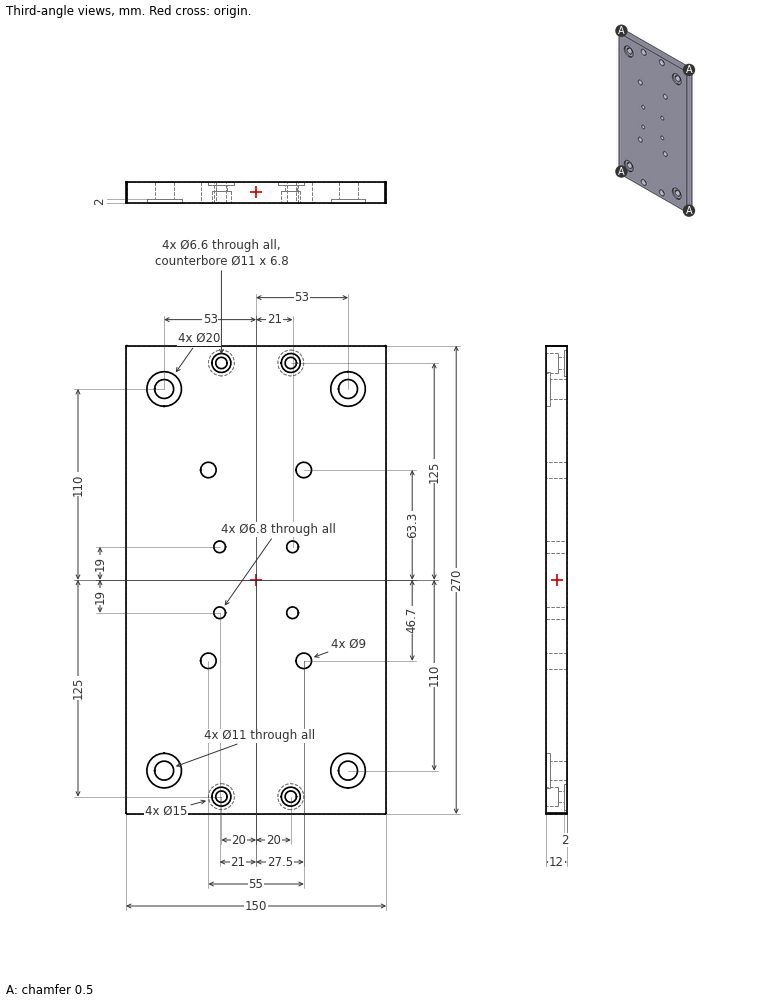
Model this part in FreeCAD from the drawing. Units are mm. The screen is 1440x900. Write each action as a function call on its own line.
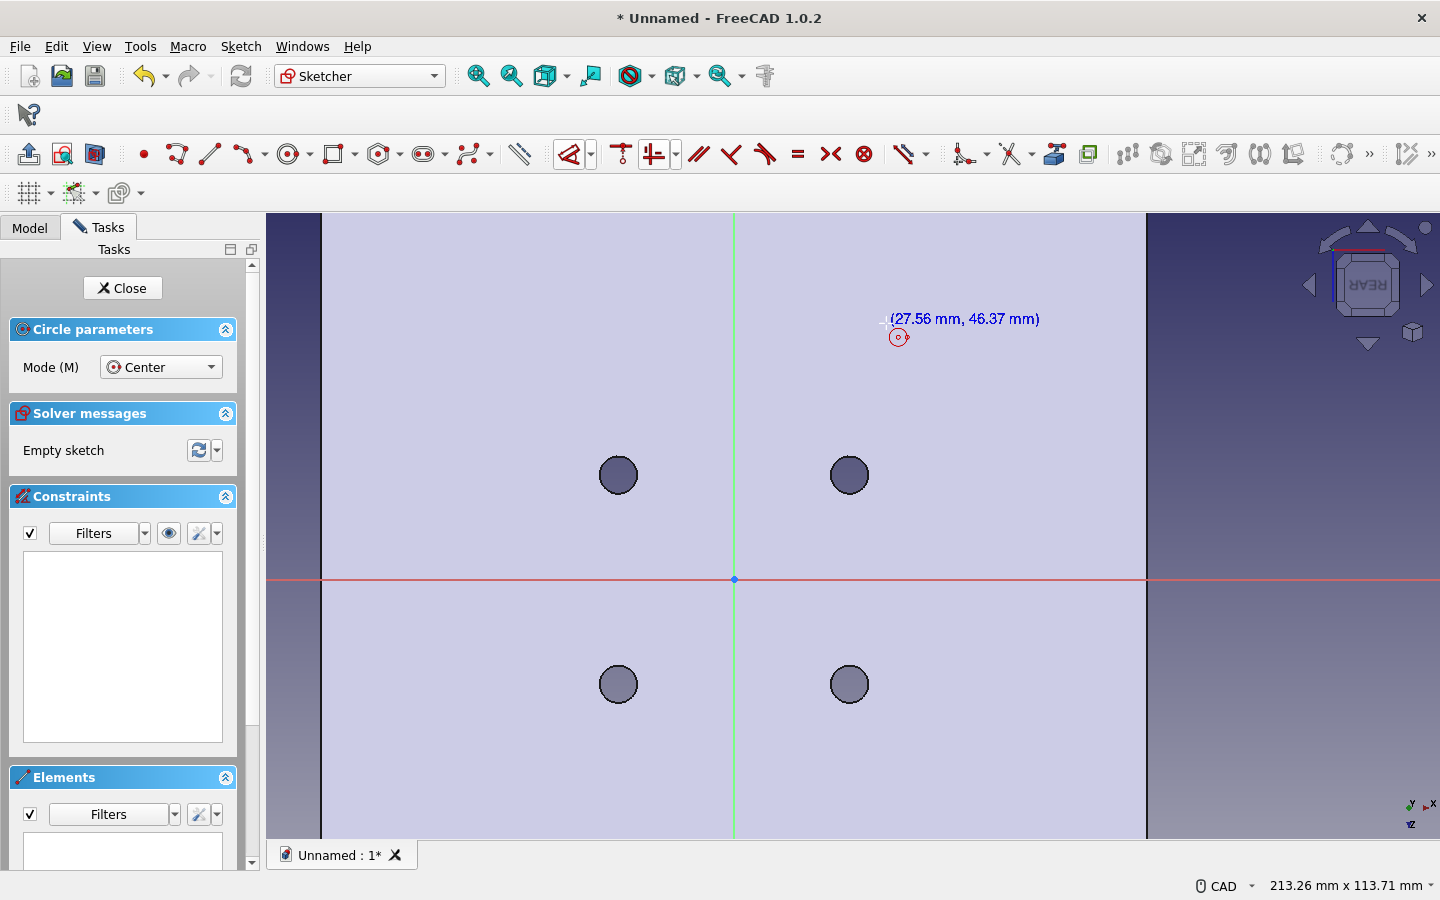
click(885, 323)
click(903, 305)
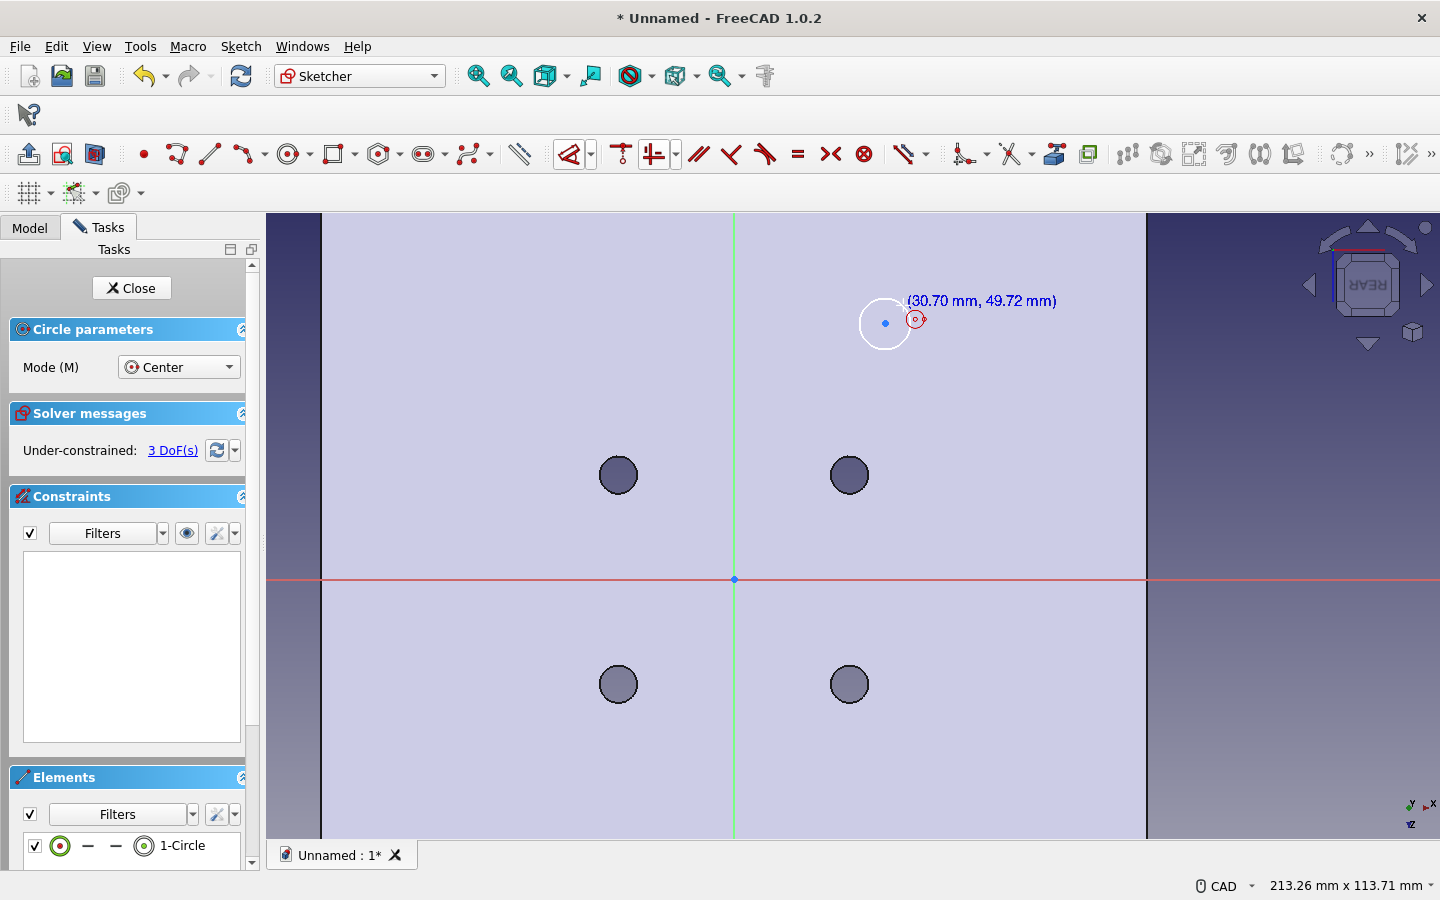
click(583, 323)
click(600, 305)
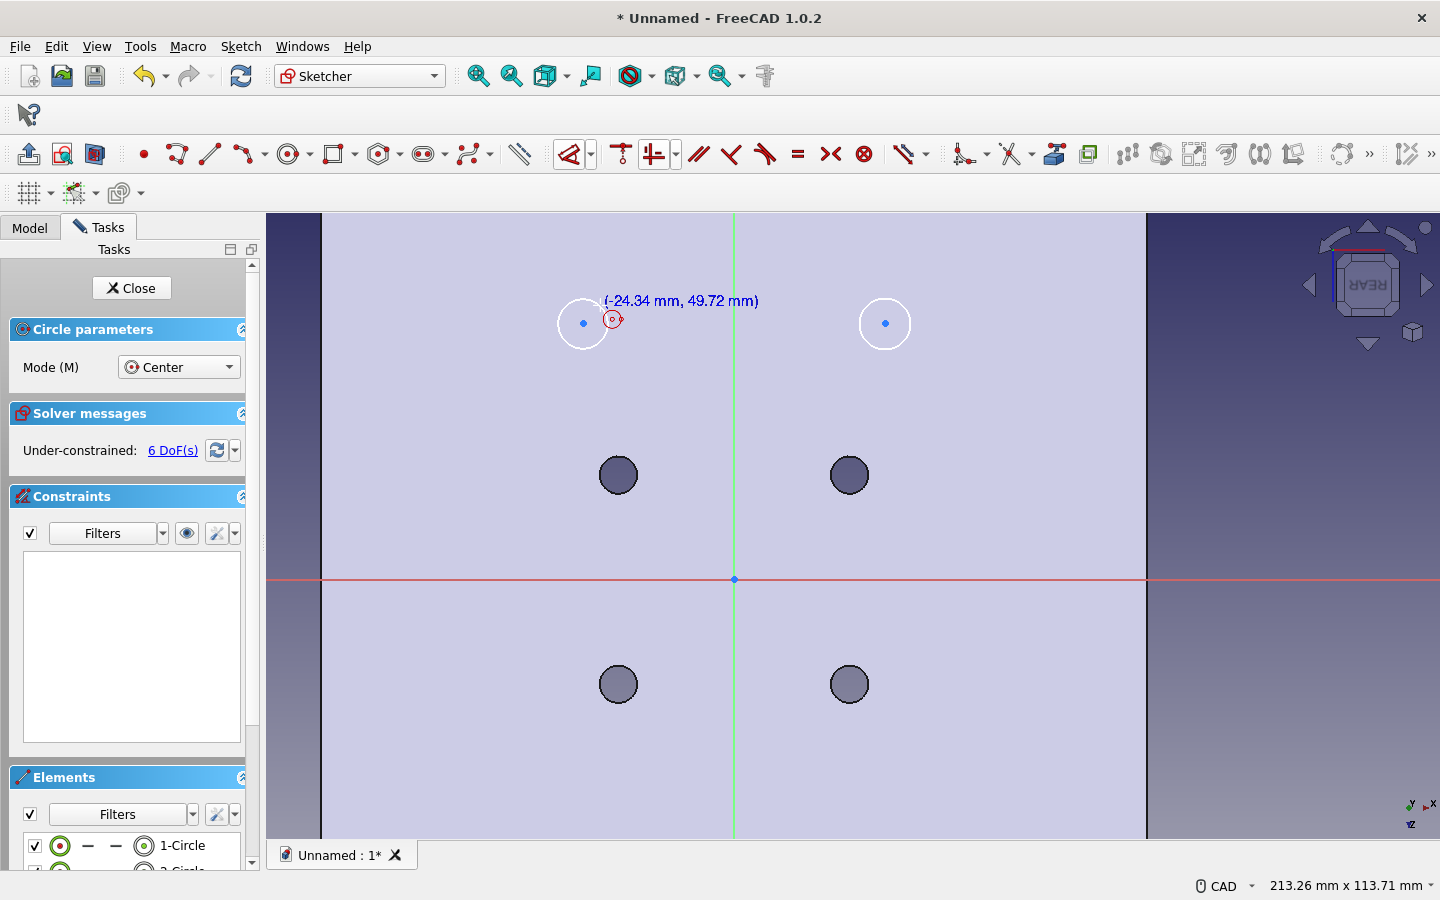
scroll(887, 324, down, 2)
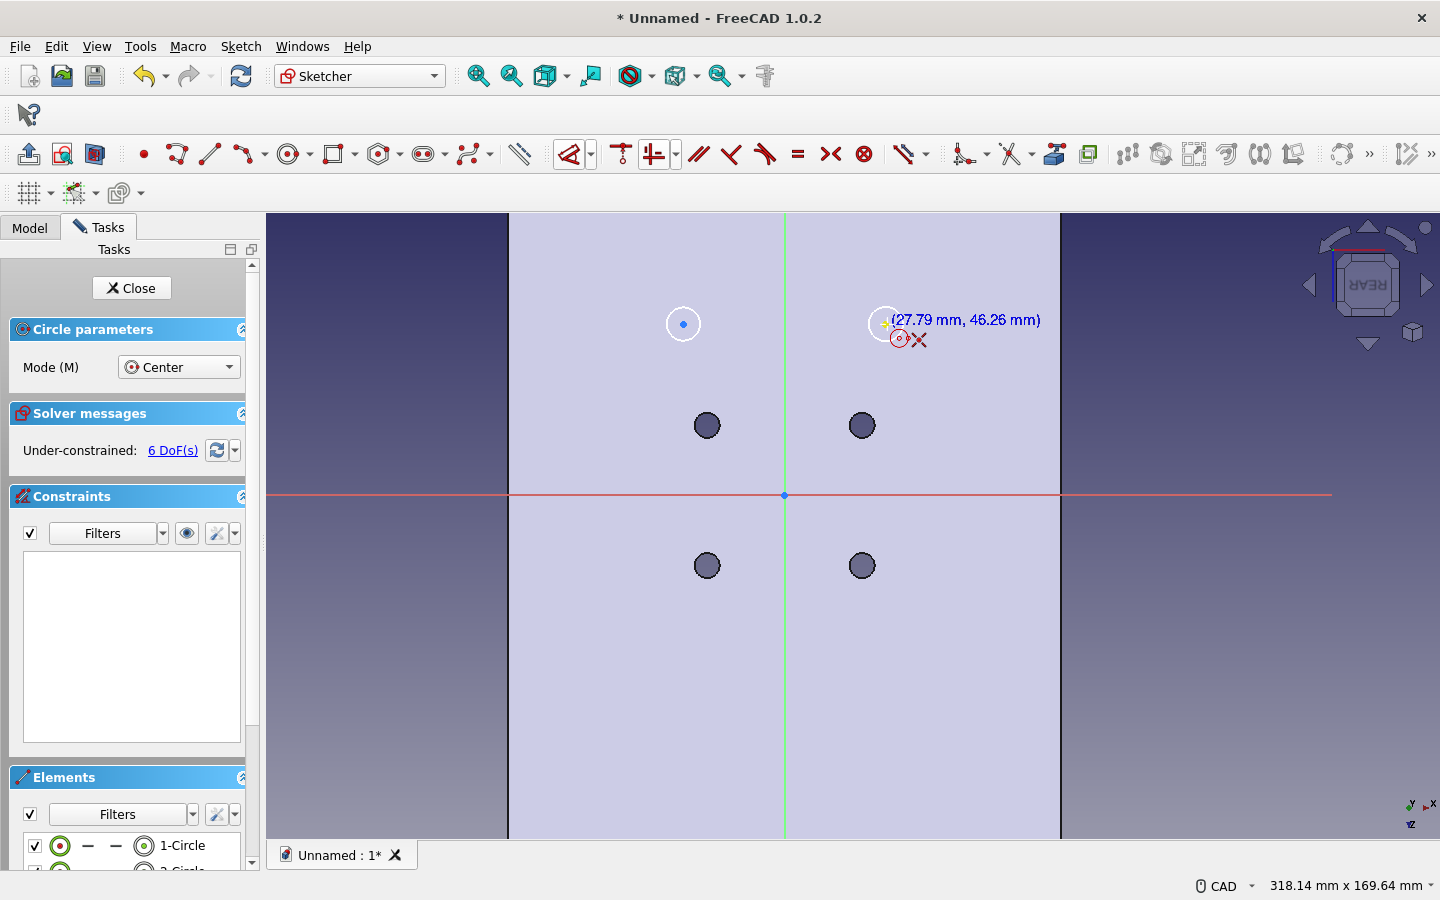
scroll(886, 729, up, 2)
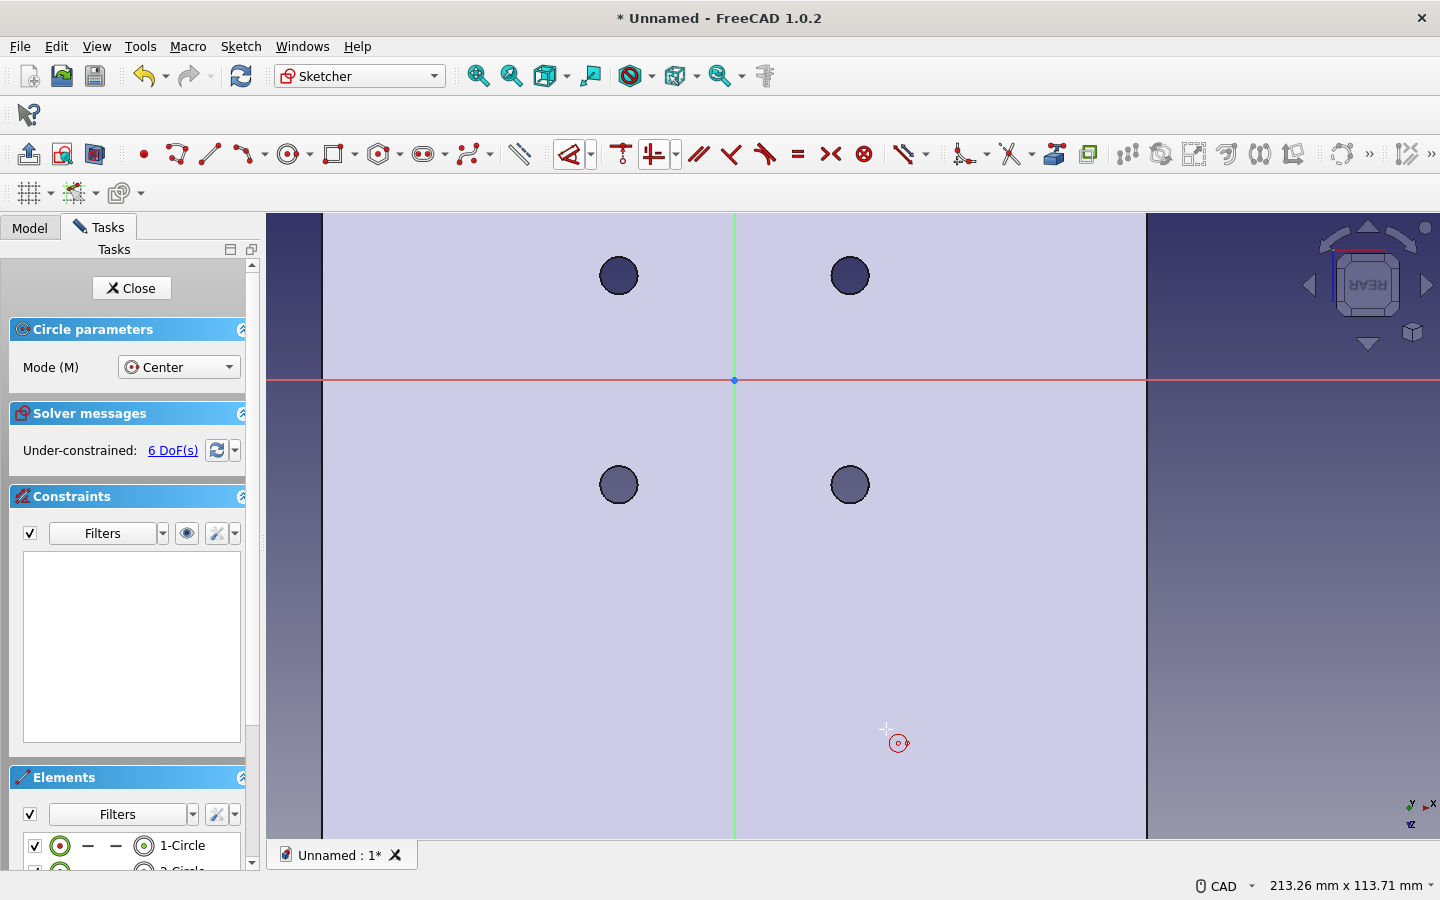
click(886, 729)
click(903, 711)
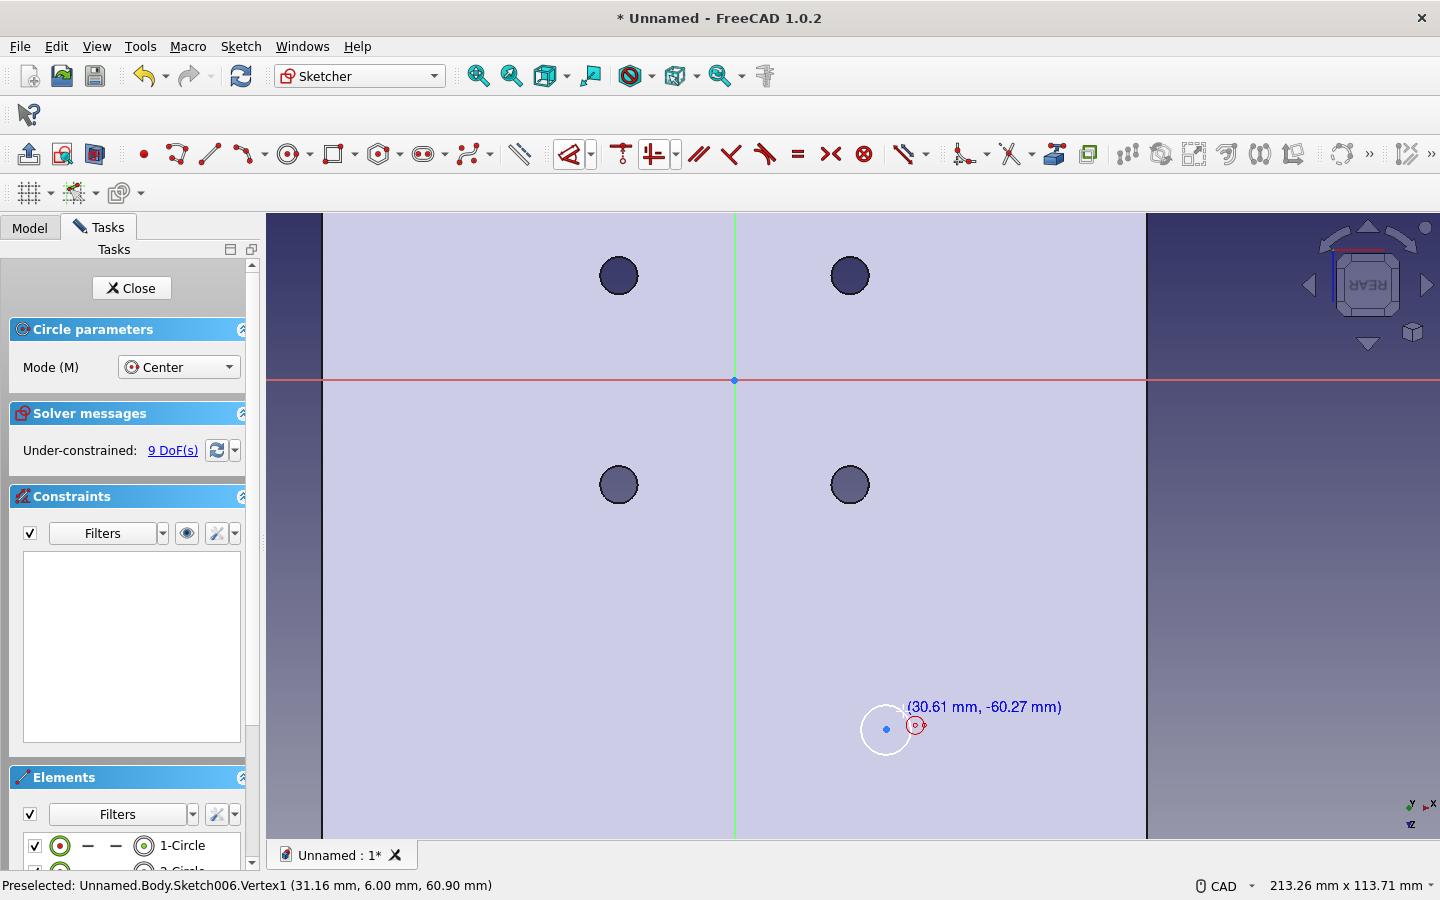
click(583, 729)
click(601, 711)
key(Escape)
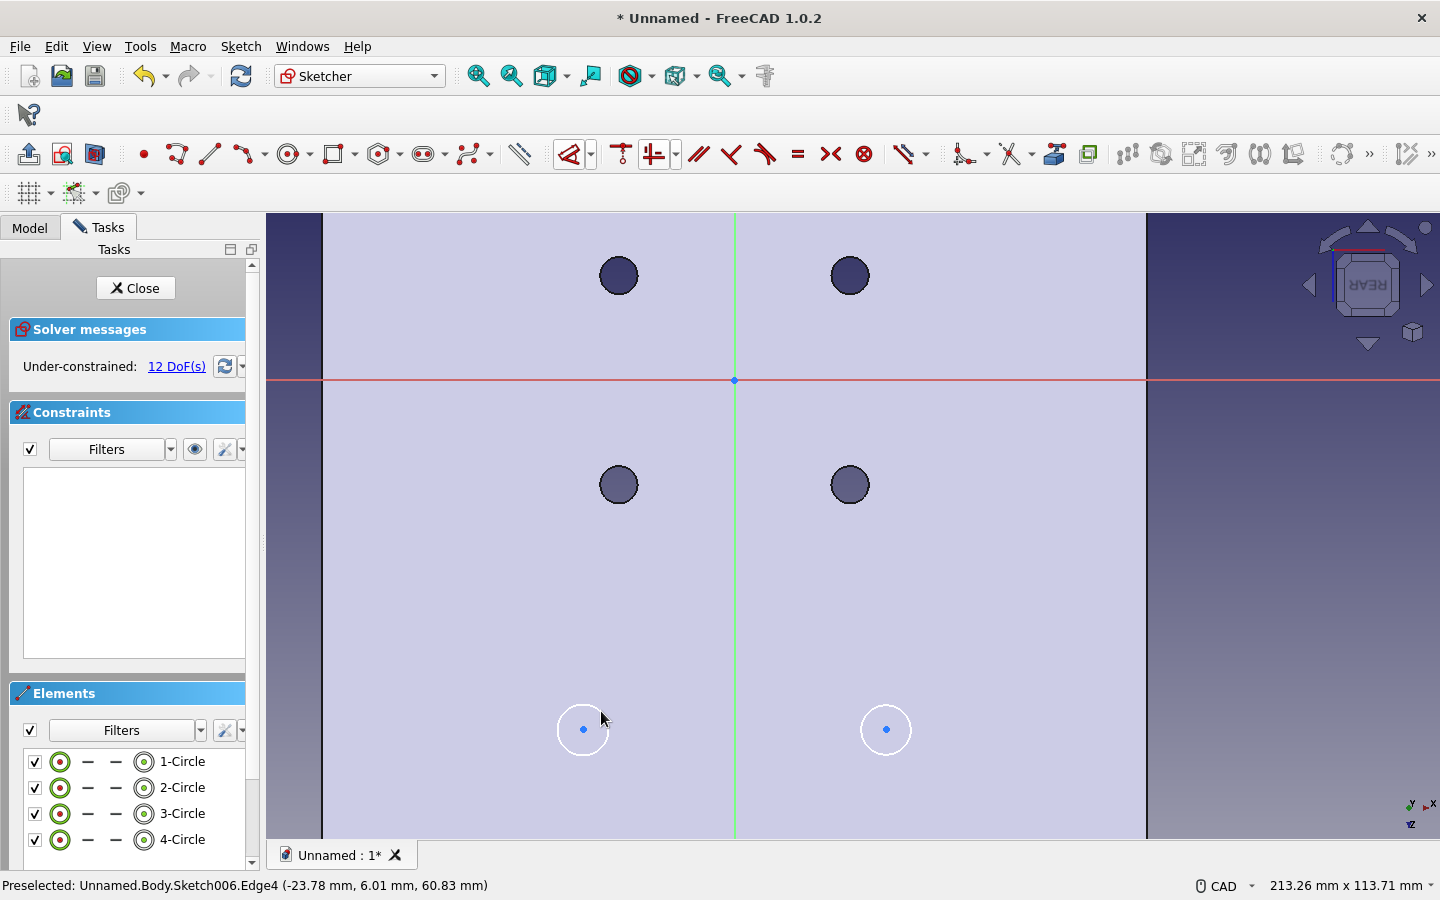
scroll(886, 730, down, 2)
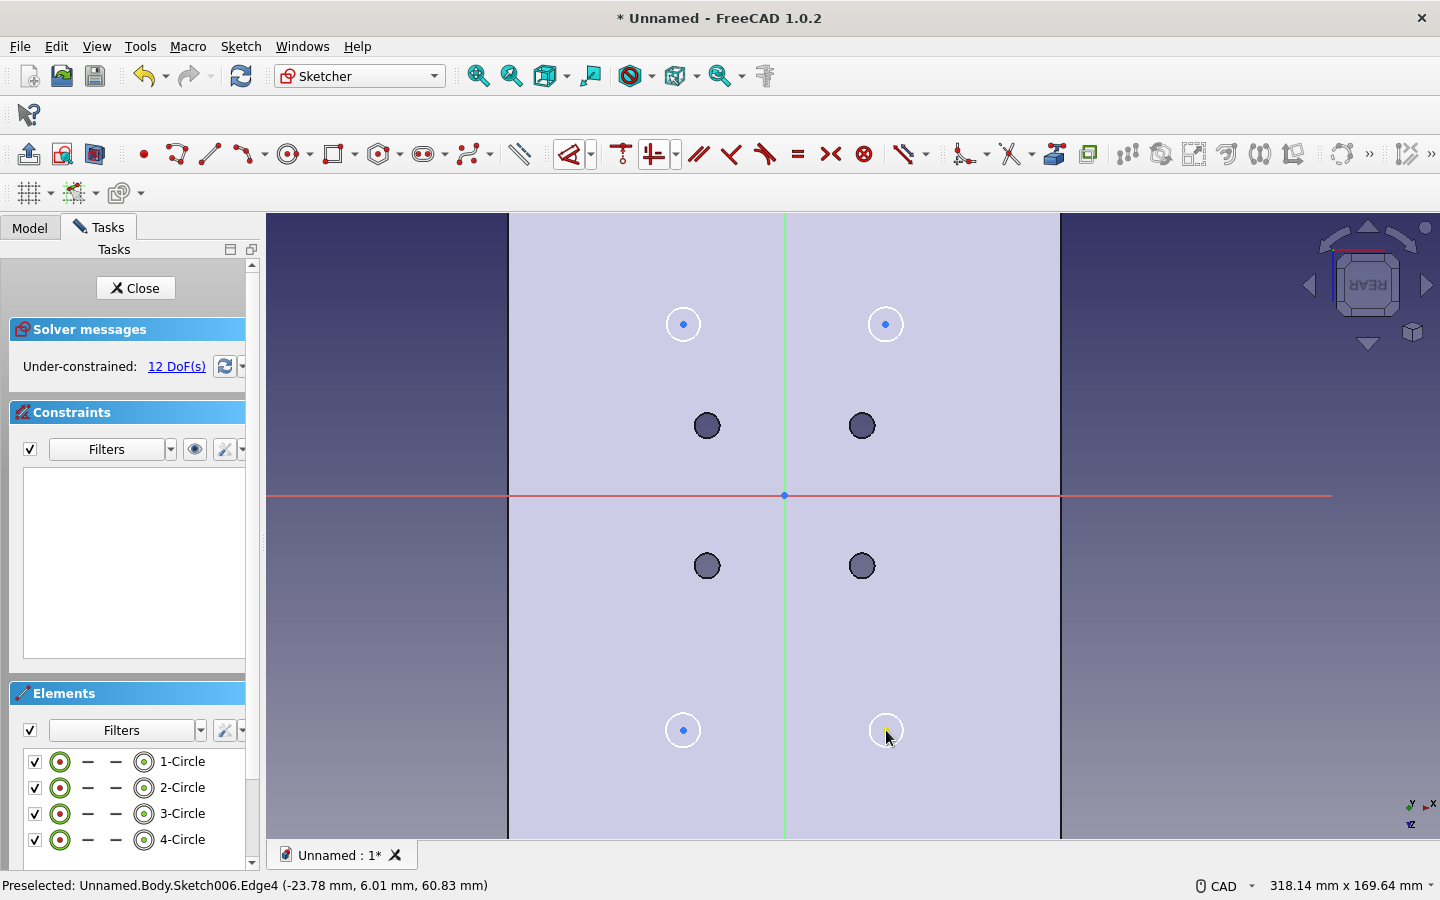
click(898, 312)